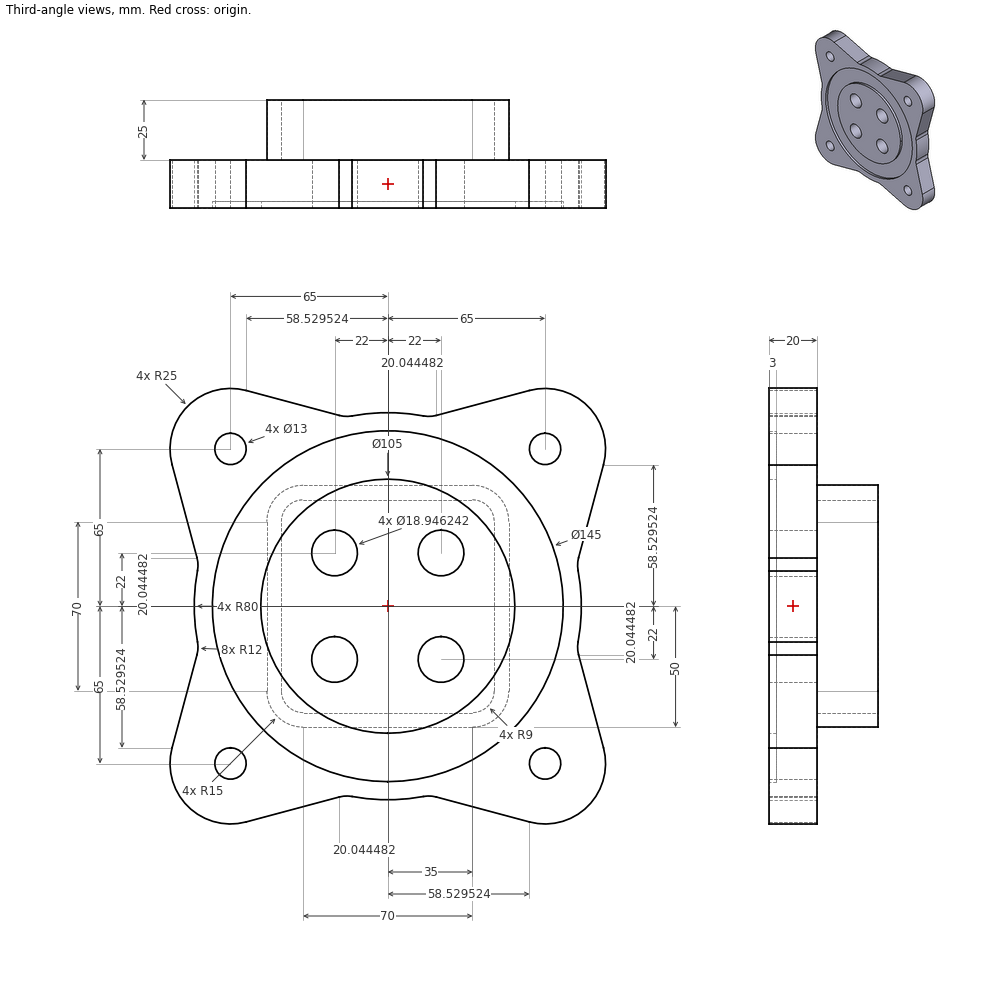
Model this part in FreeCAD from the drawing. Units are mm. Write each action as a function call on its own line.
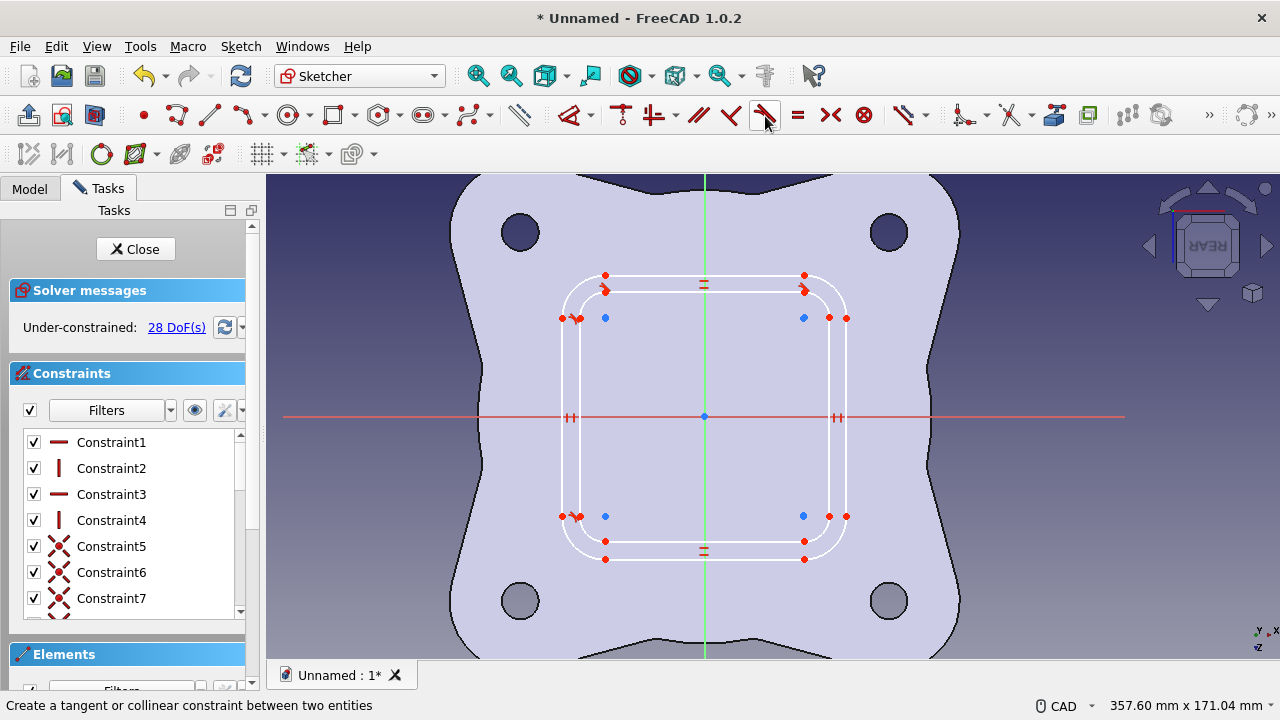
click(665, 560)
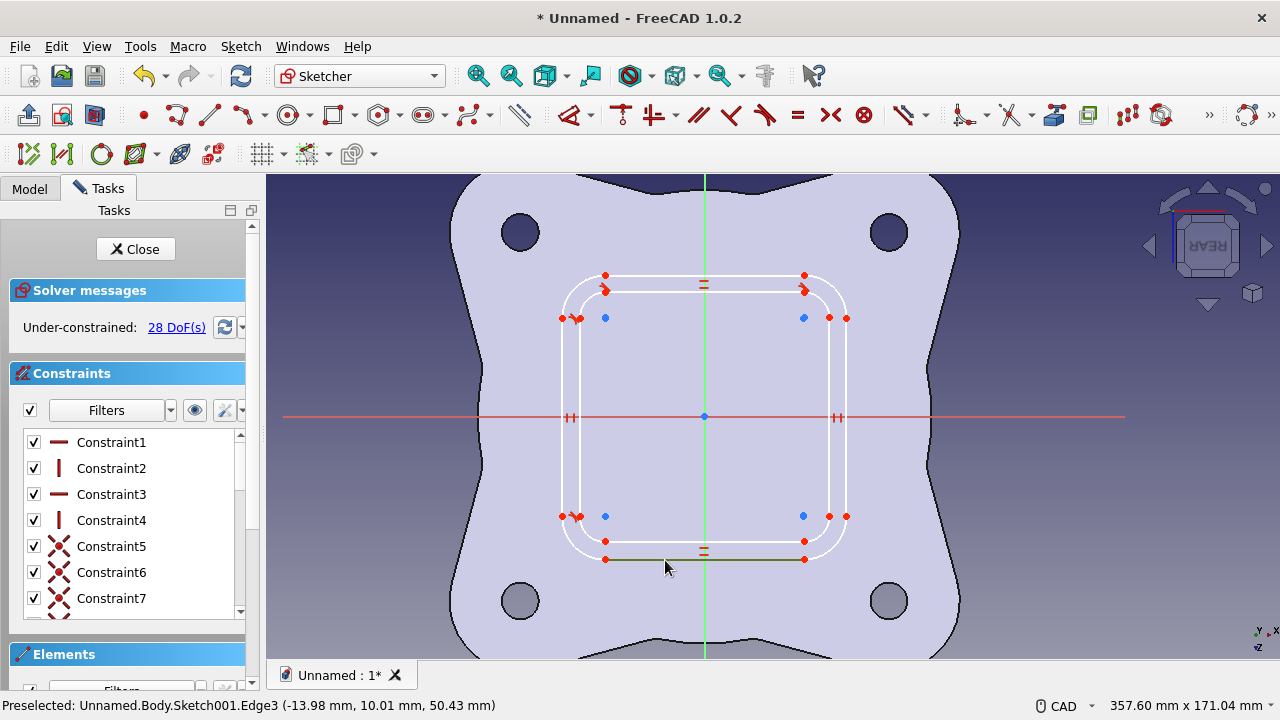
click(567, 536)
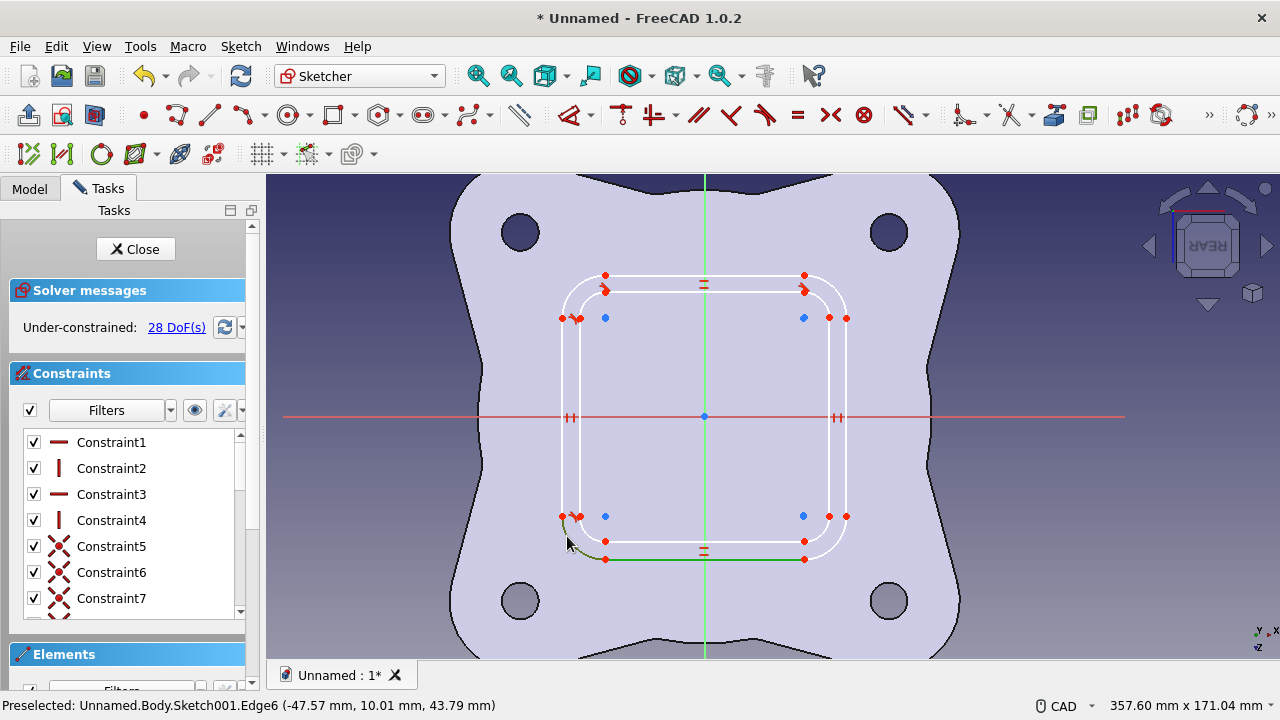
click(765, 116)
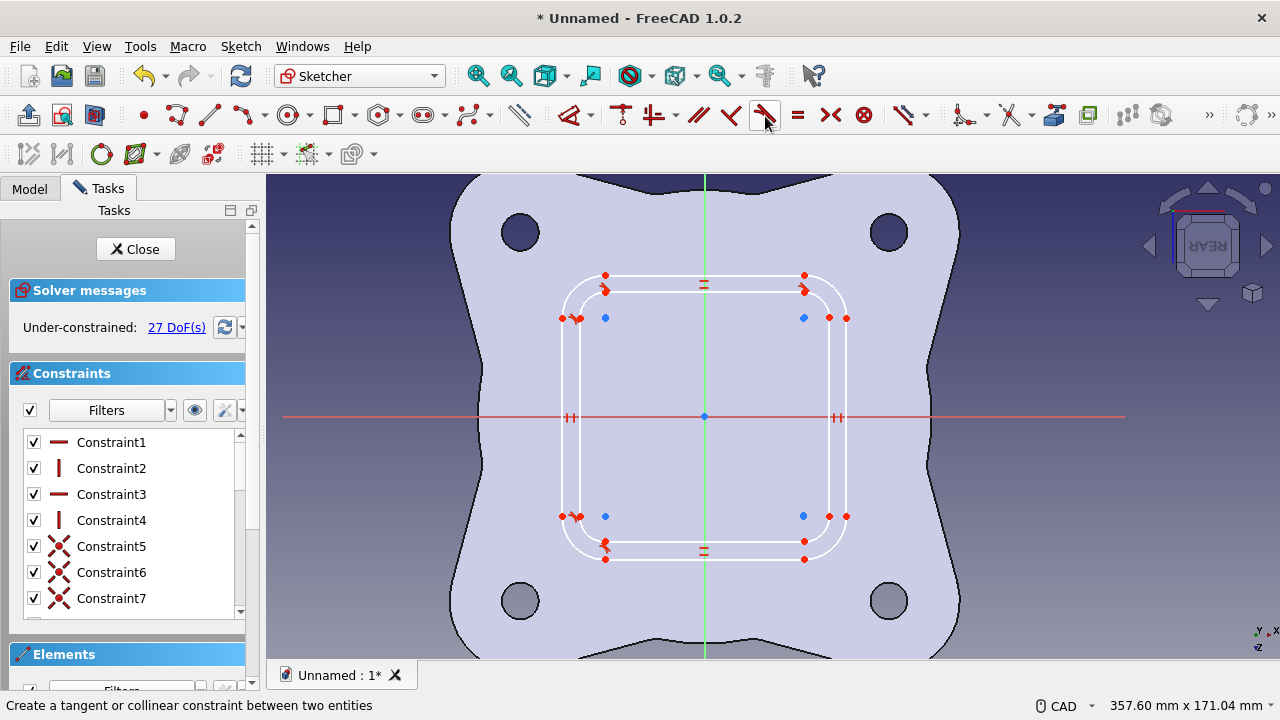
click(665, 560)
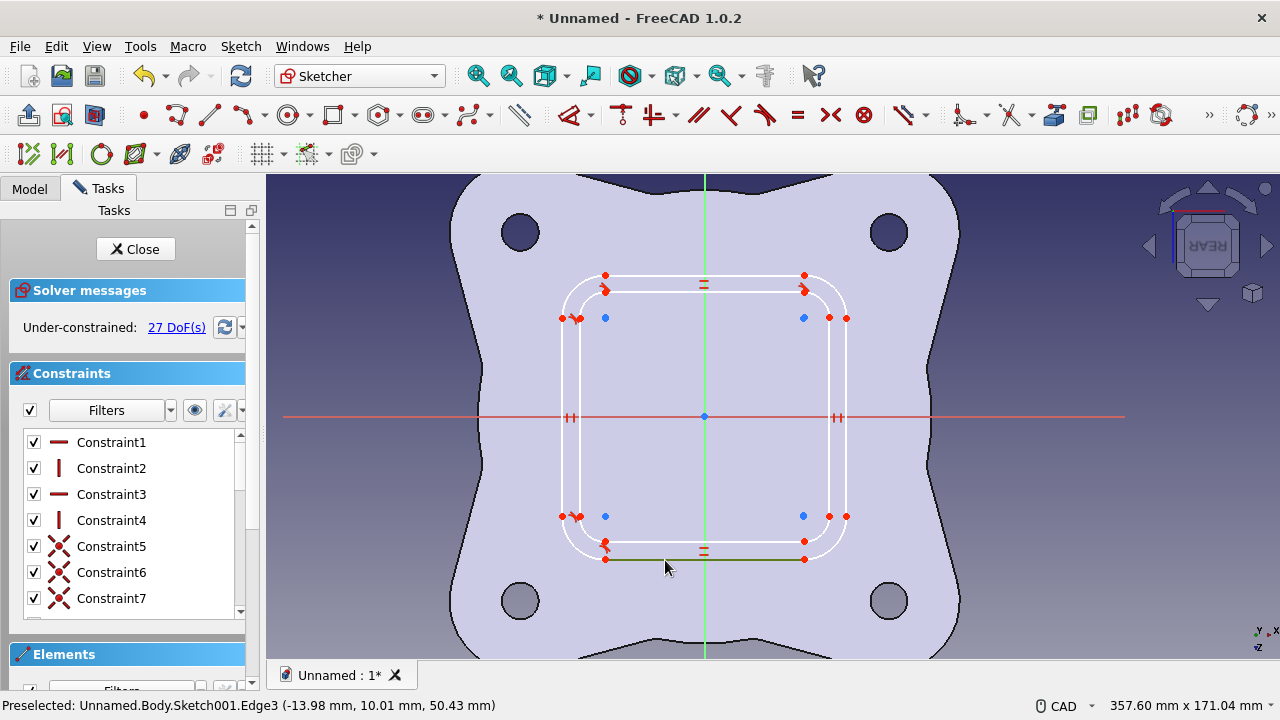
click(823, 555)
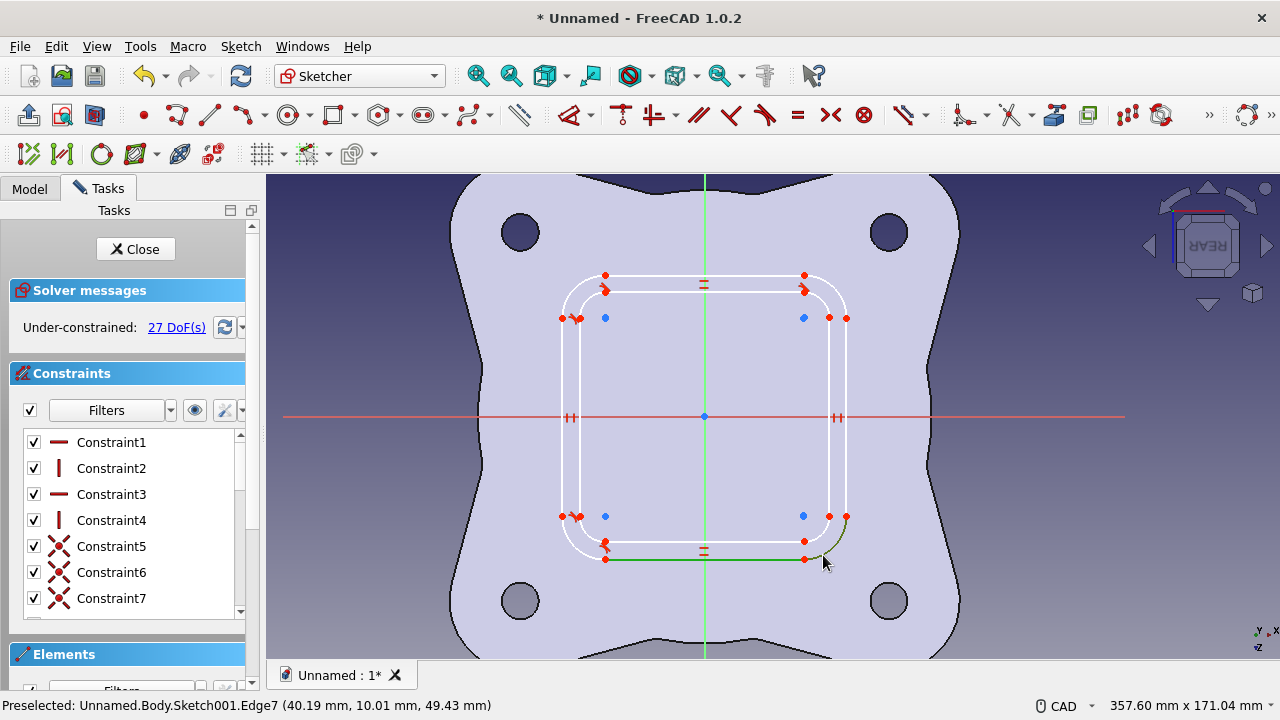
click(765, 116)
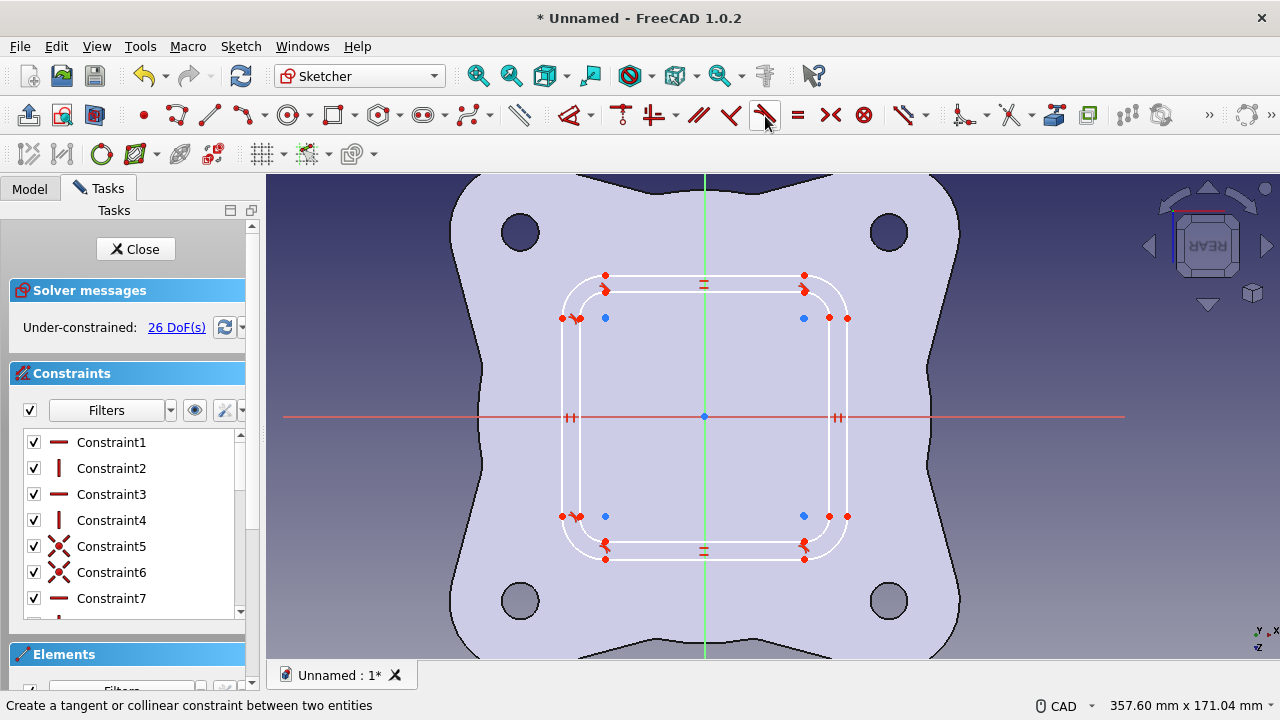
click(847, 457)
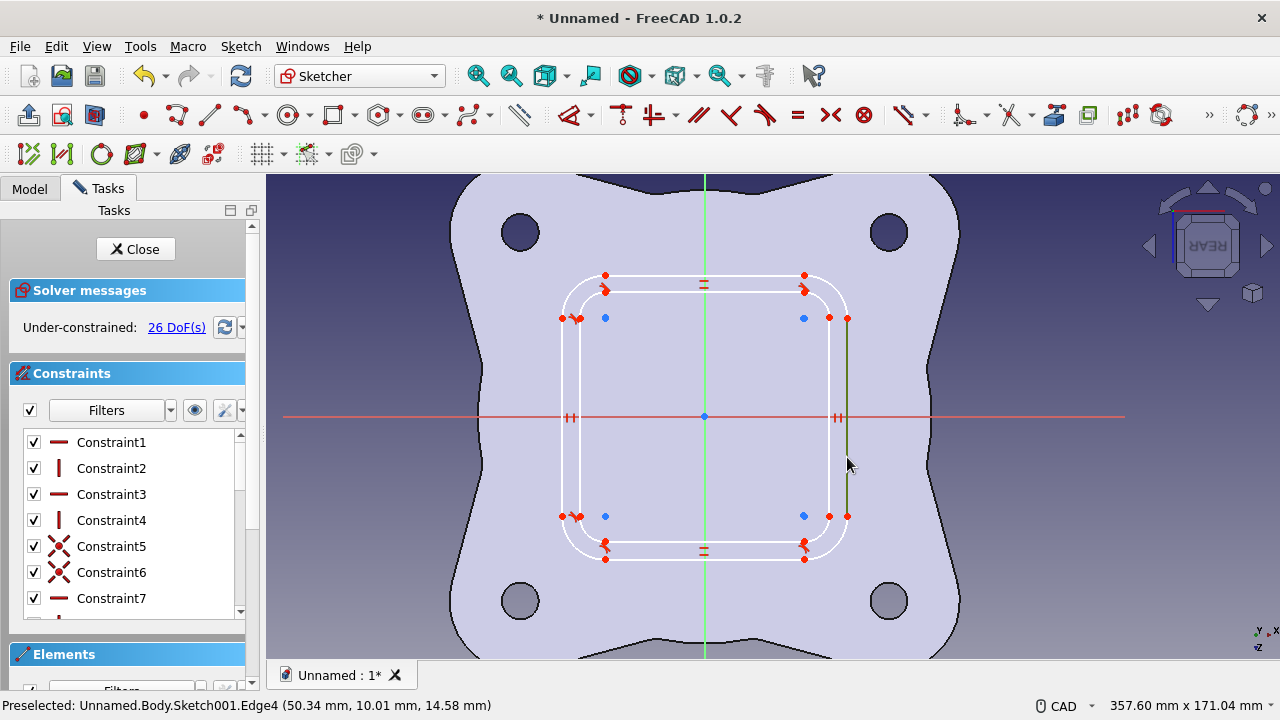
click(824, 555)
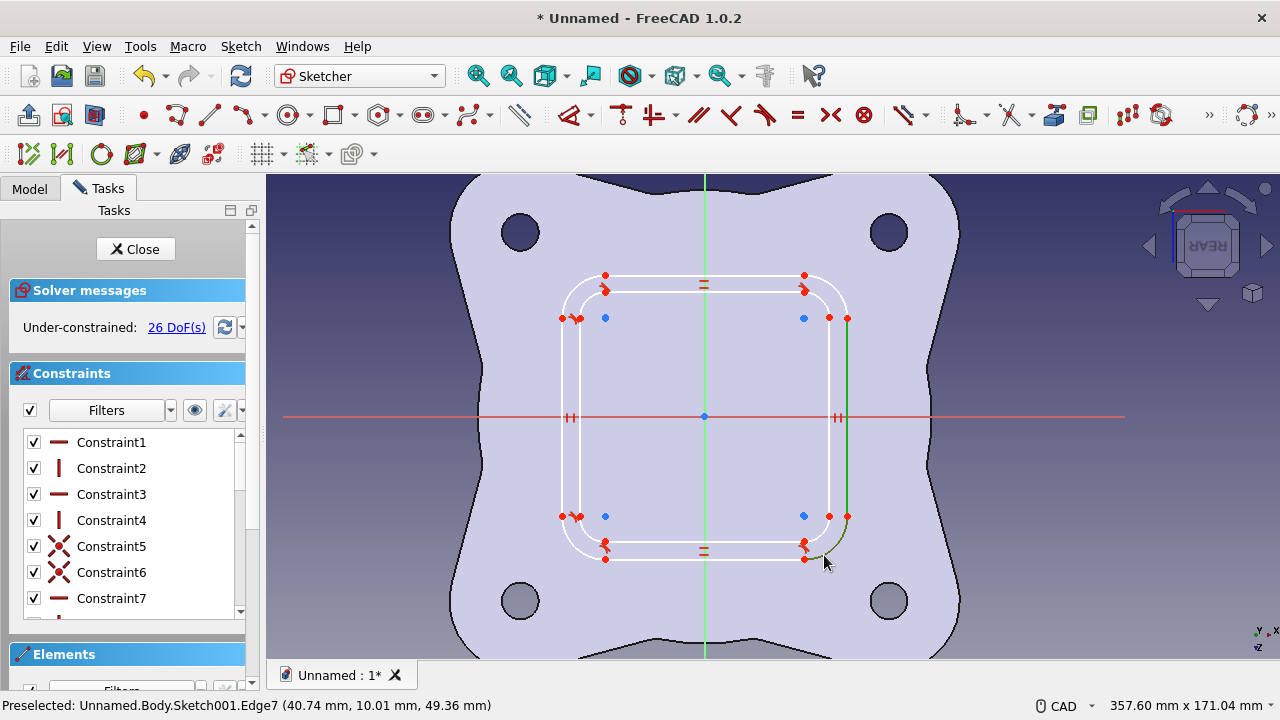
click(765, 116)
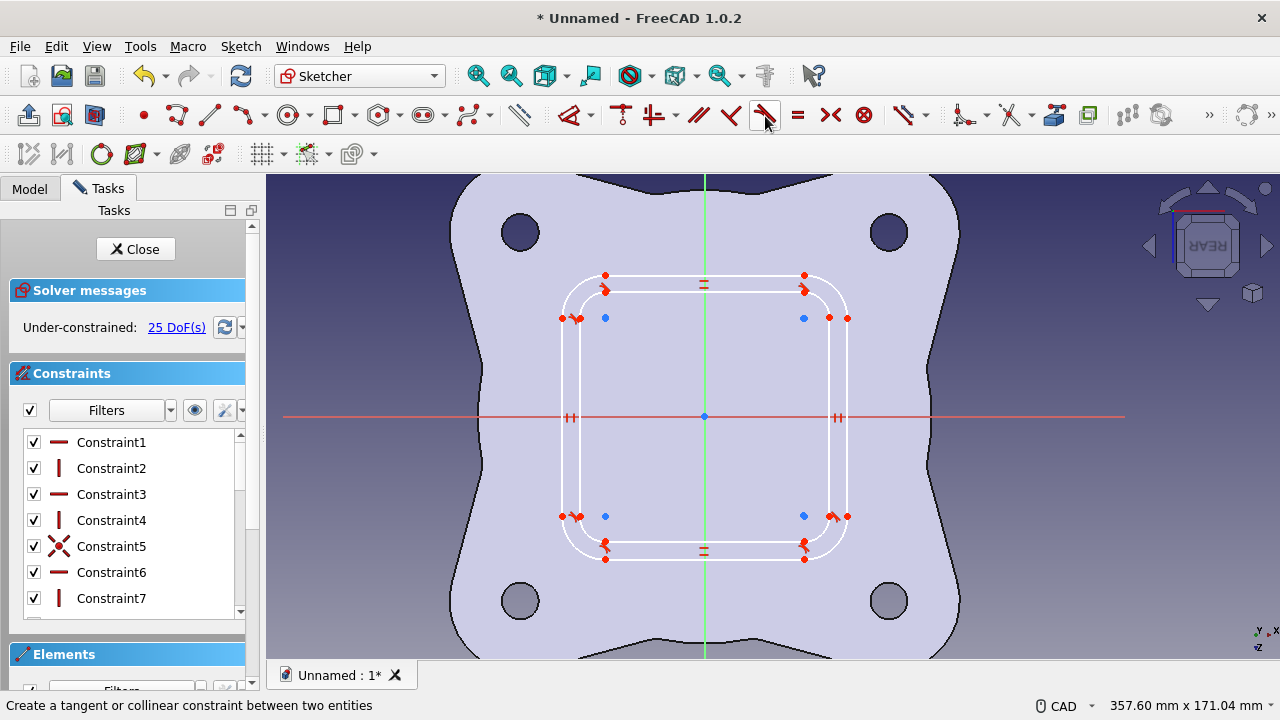
click(847, 457)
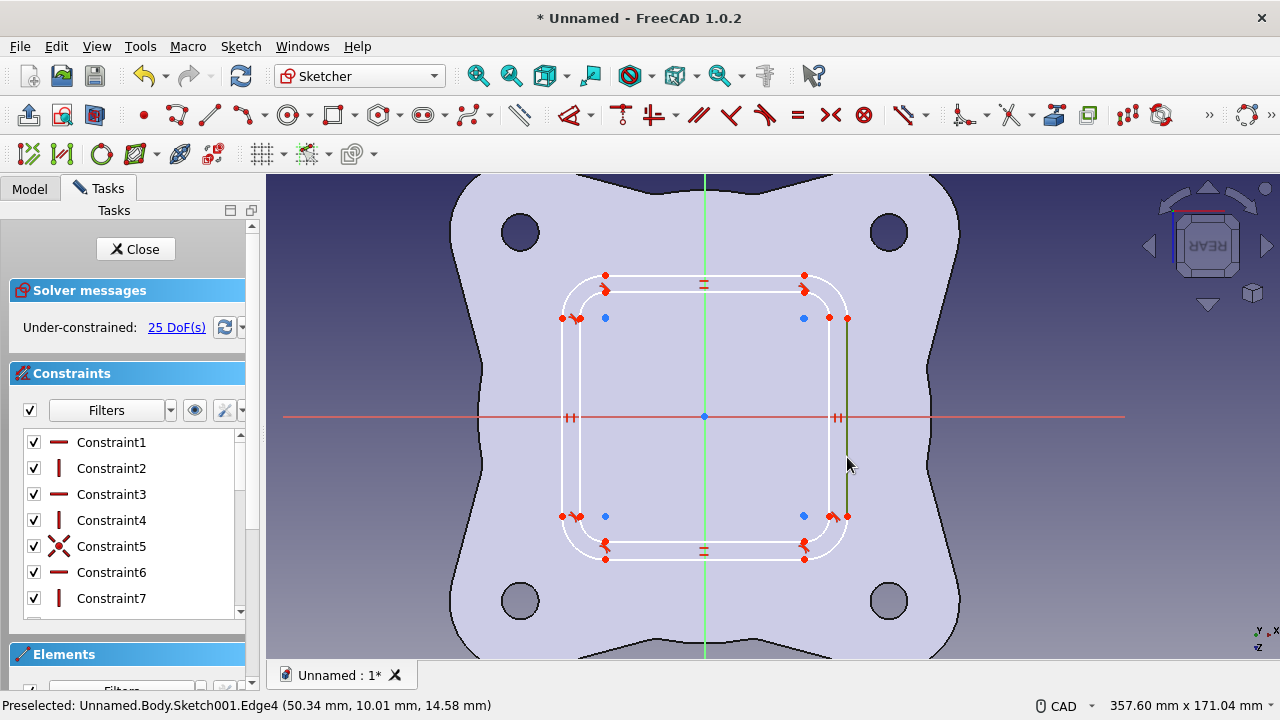
click(843, 299)